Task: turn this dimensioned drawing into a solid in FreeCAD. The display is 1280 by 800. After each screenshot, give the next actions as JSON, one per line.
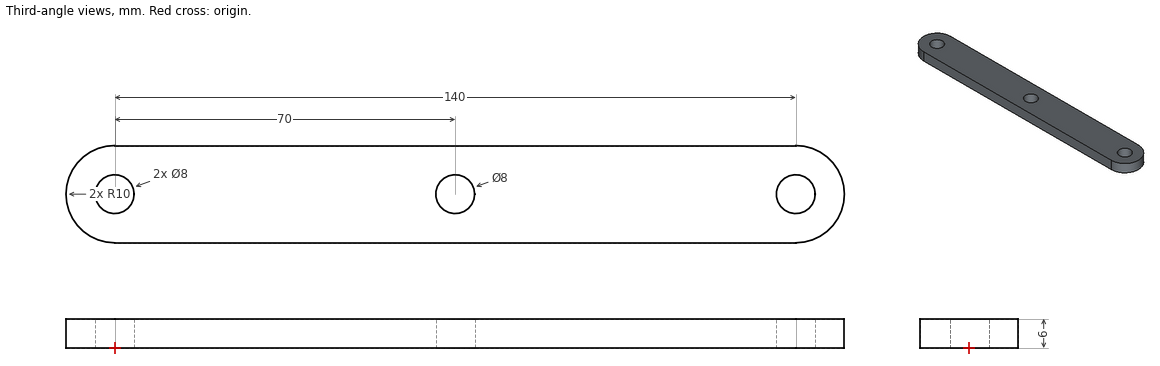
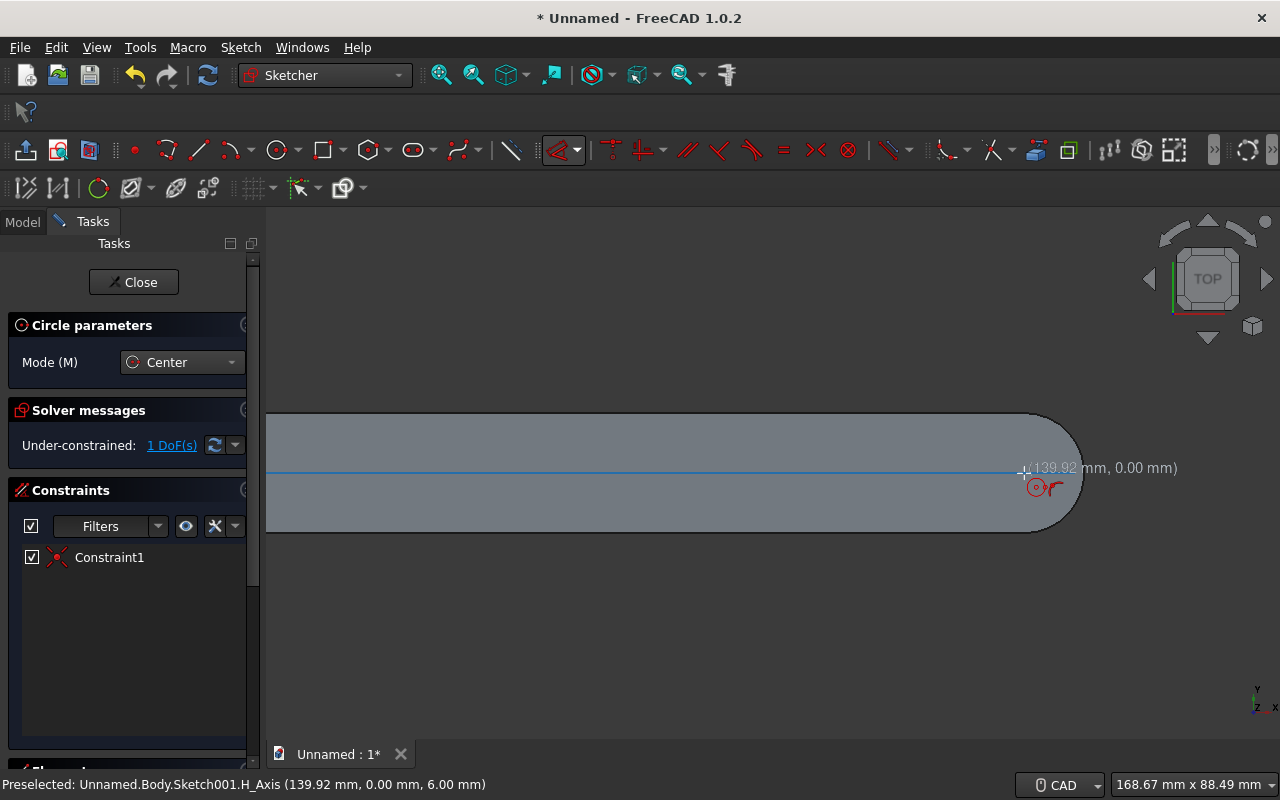
{"action": "left_click", "coordinate": [1024, 473]}
{"action": "left_click", "coordinate": [1041, 456]}
{"action": "key", "text": "Escape"}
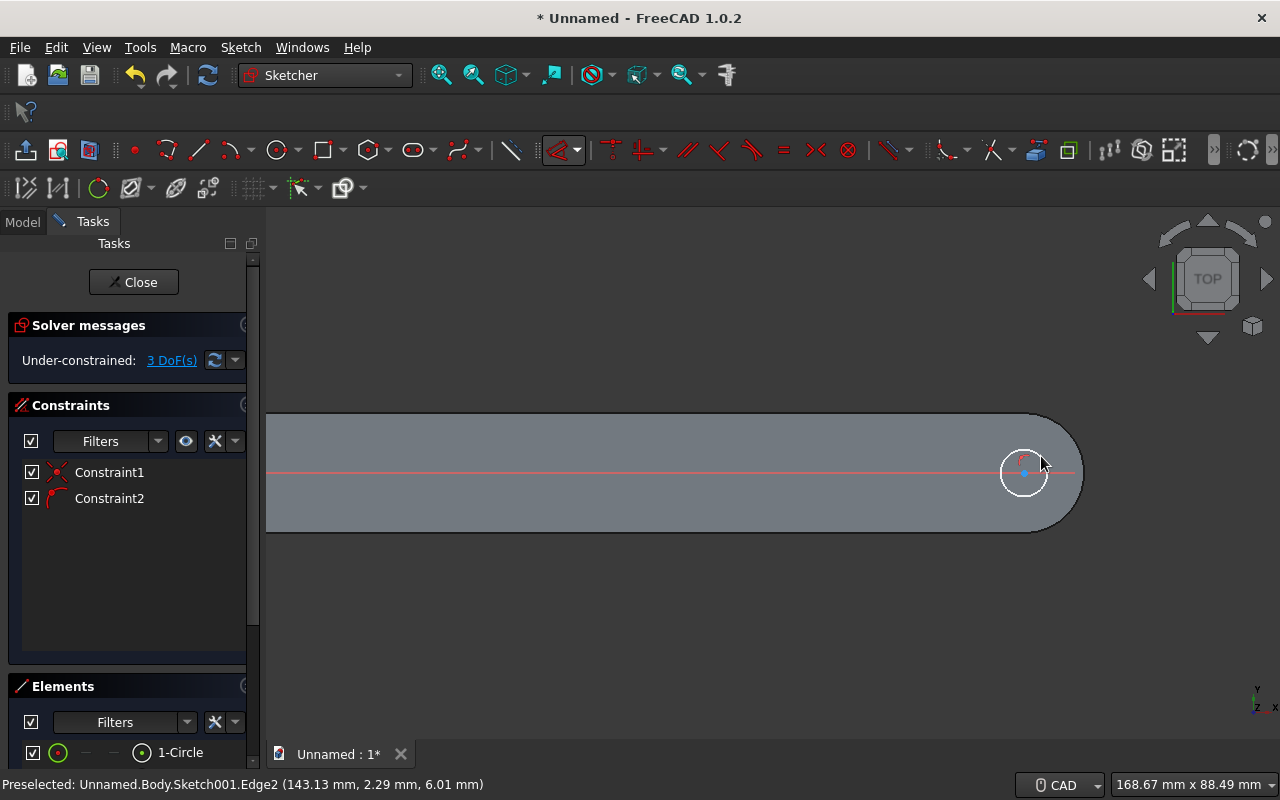
{"action": "scroll", "coordinate": [910, 473], "scroll_direction": "down", "scroll_amount": 2}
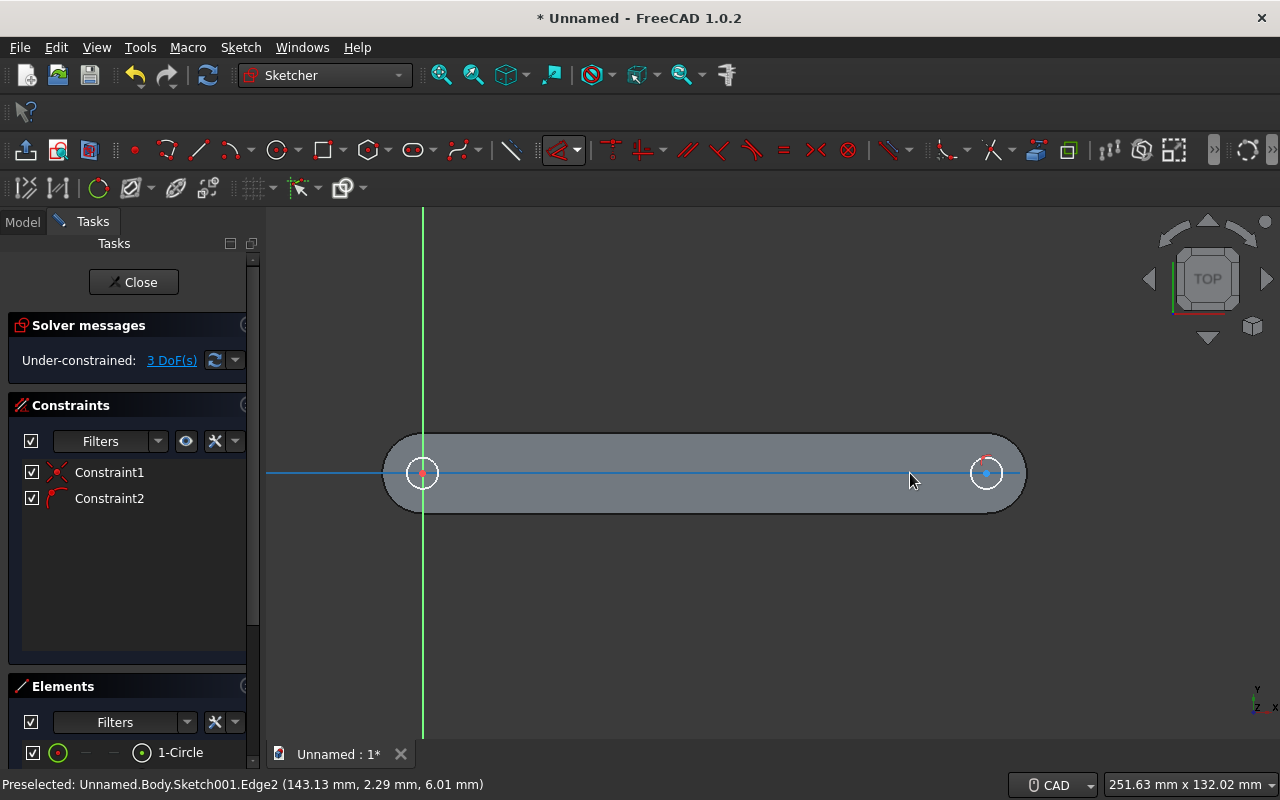
{"action": "scroll", "coordinate": [433, 462], "scroll_direction": "up", "scroll_amount": 2}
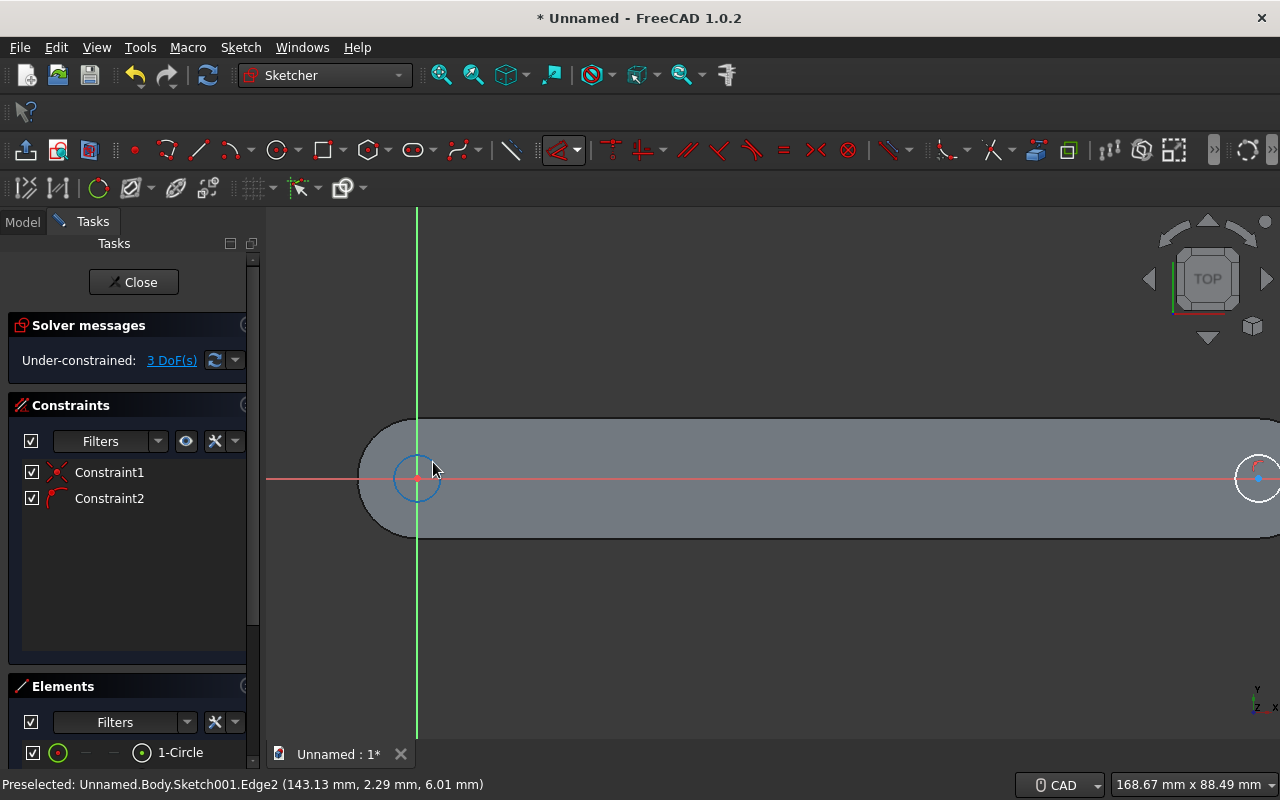
{"action": "left_click", "coordinate": [434, 462]}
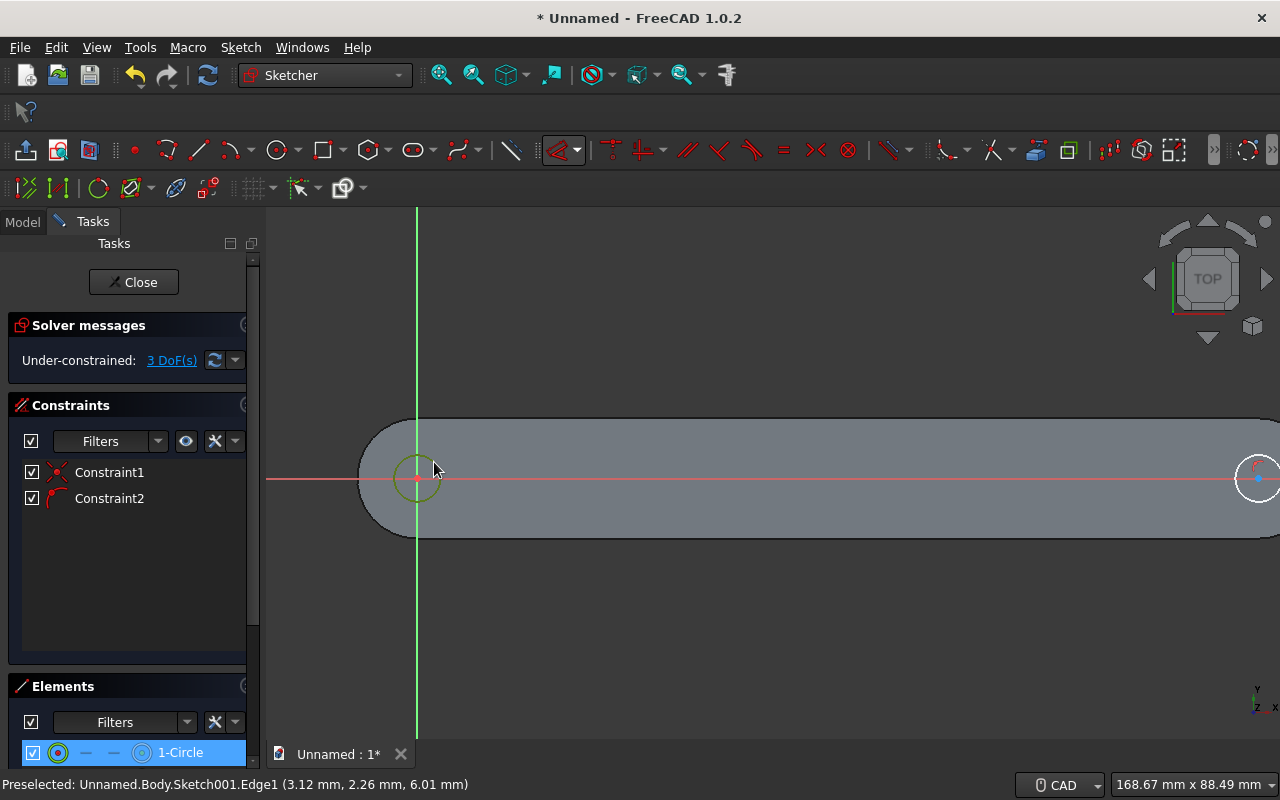
{"action": "scroll", "coordinate": [433, 462], "scroll_direction": "down", "scroll_amount": 2}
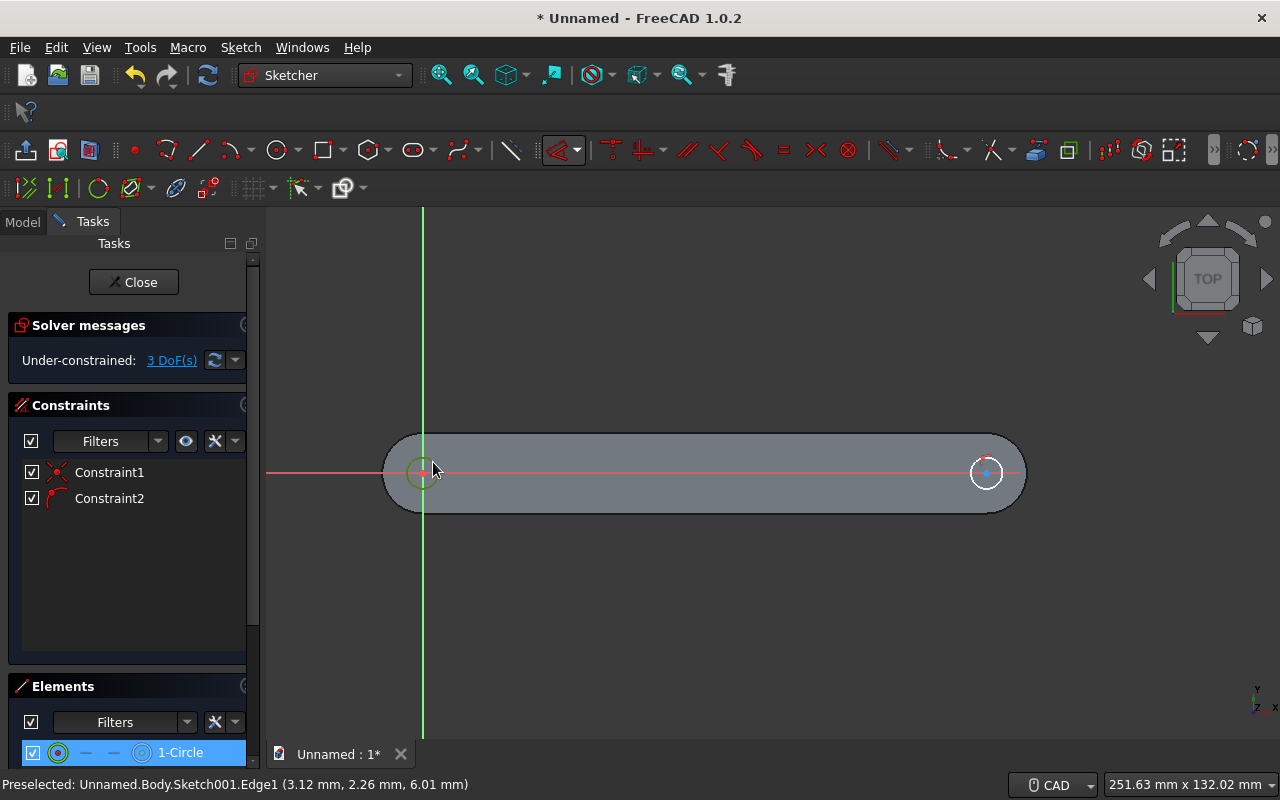
{"action": "scroll", "coordinate": [998, 462], "scroll_direction": "up", "scroll_amount": 2}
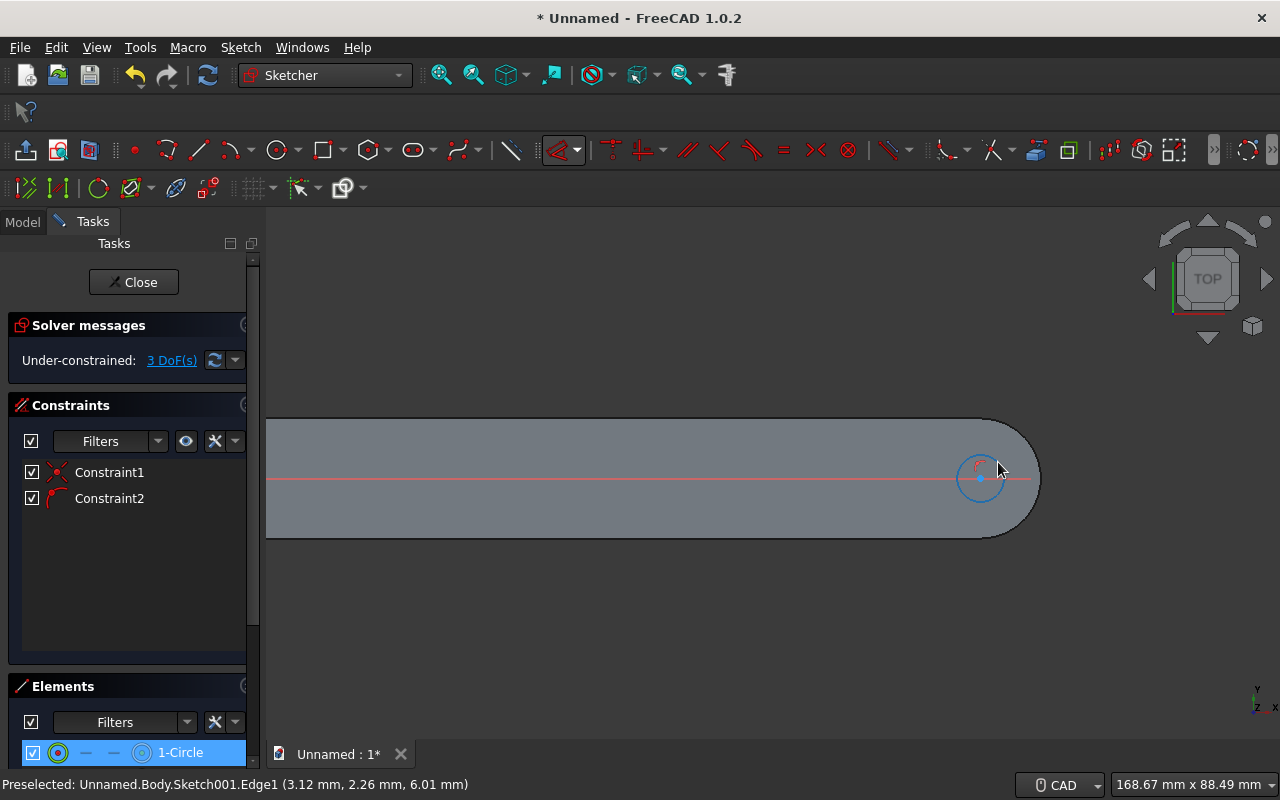
{"action": "left_click", "coordinate": [997, 462]}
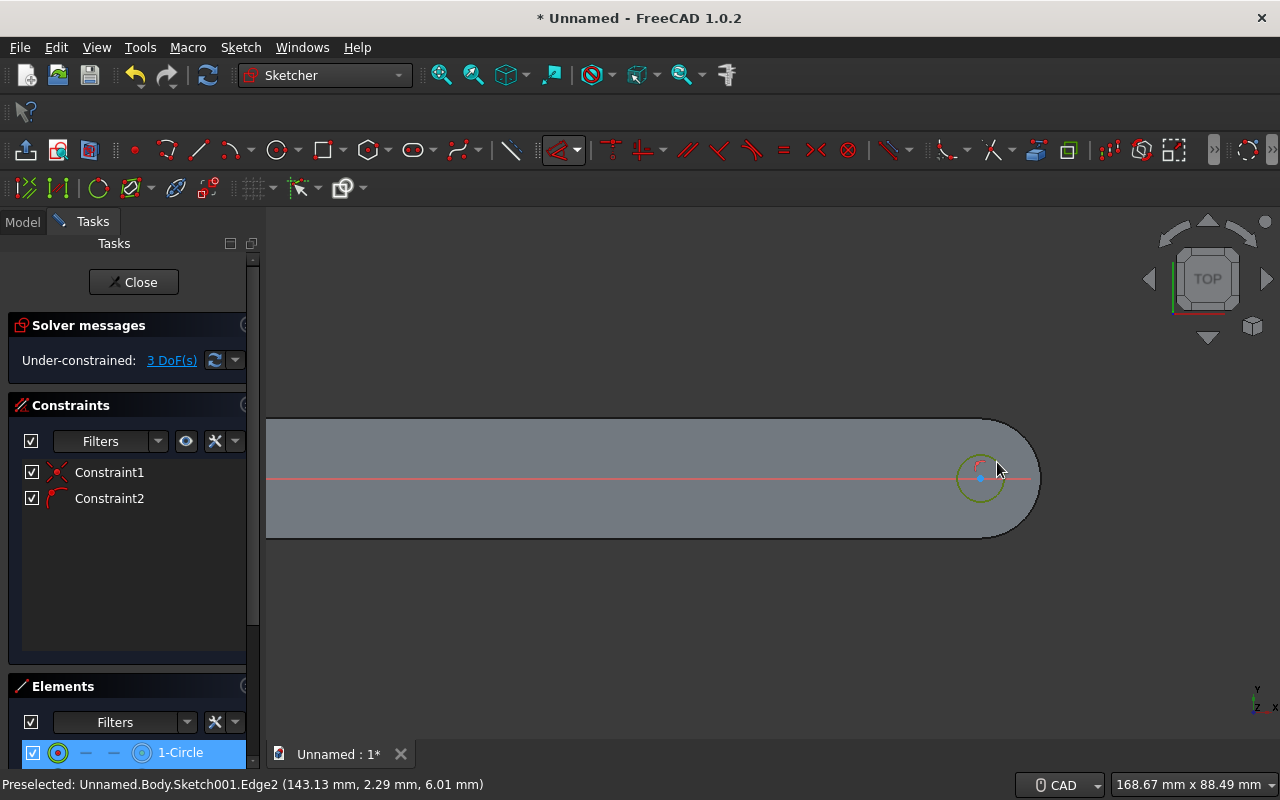
{"action": "left_click", "coordinate": [784, 150]}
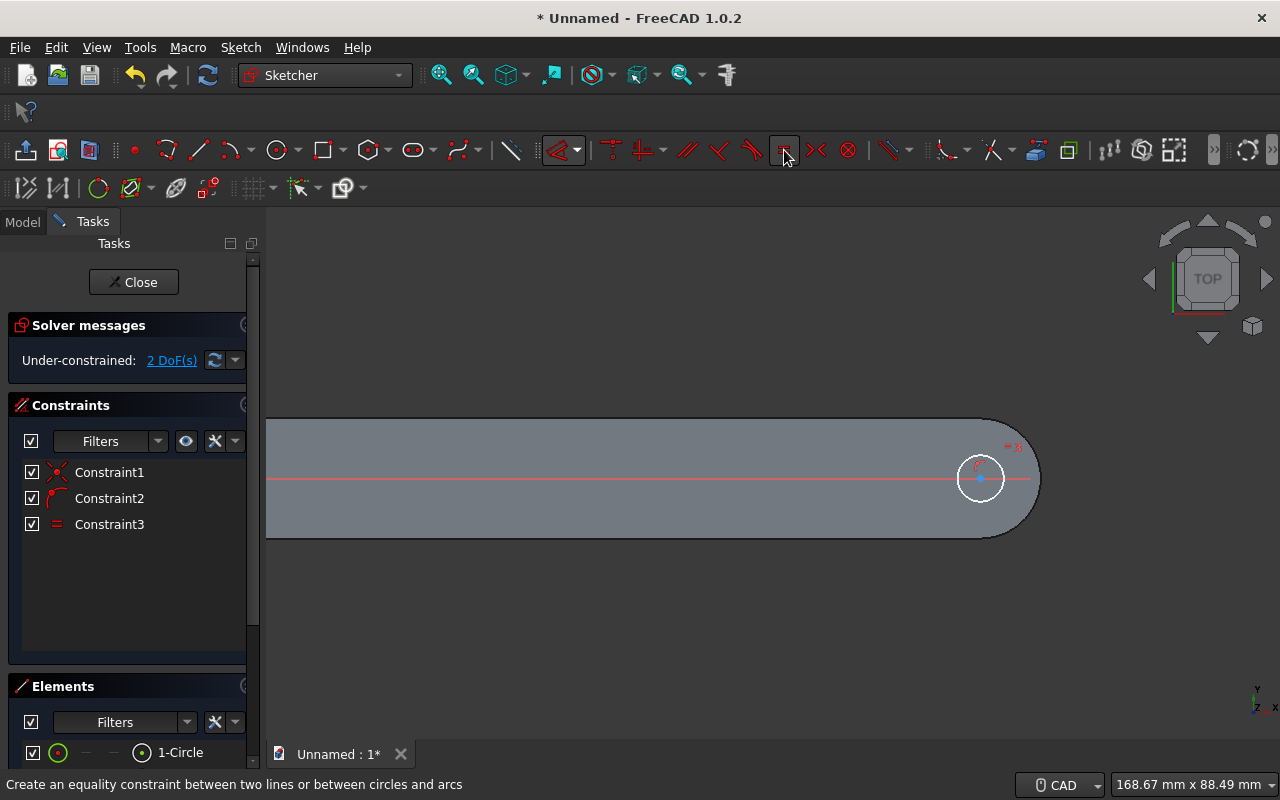
{"action": "scroll", "coordinate": [998, 462], "scroll_direction": "down", "scroll_amount": 2}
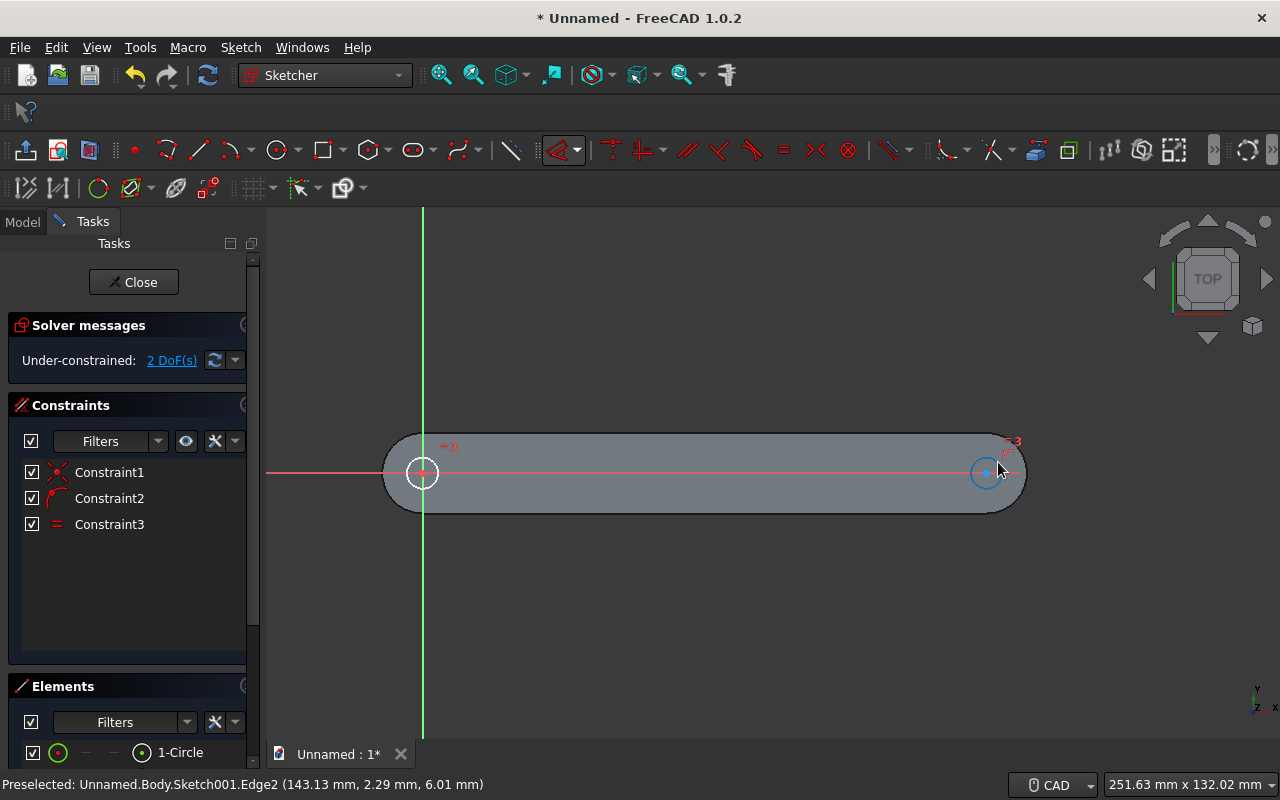
{"action": "scroll", "coordinate": [433, 462], "scroll_direction": "up", "scroll_amount": 2}